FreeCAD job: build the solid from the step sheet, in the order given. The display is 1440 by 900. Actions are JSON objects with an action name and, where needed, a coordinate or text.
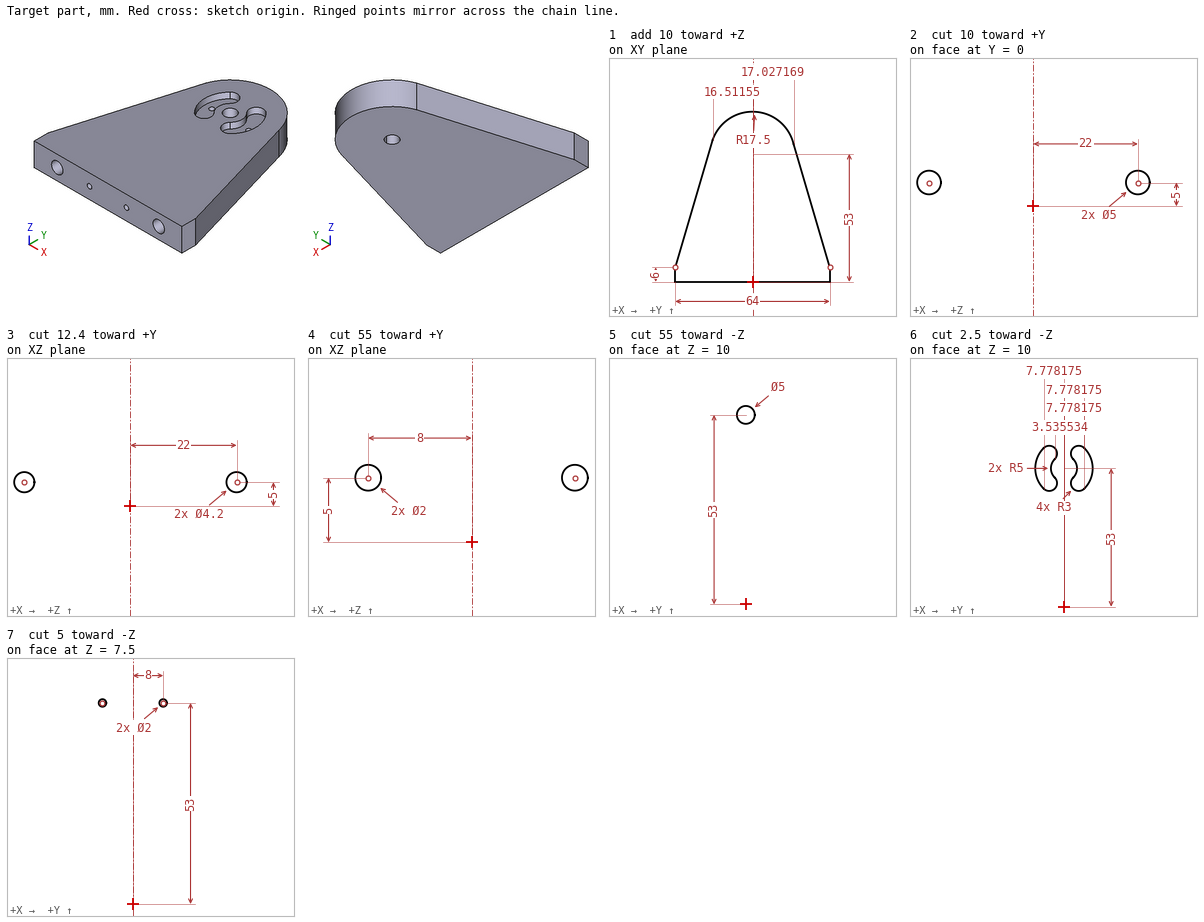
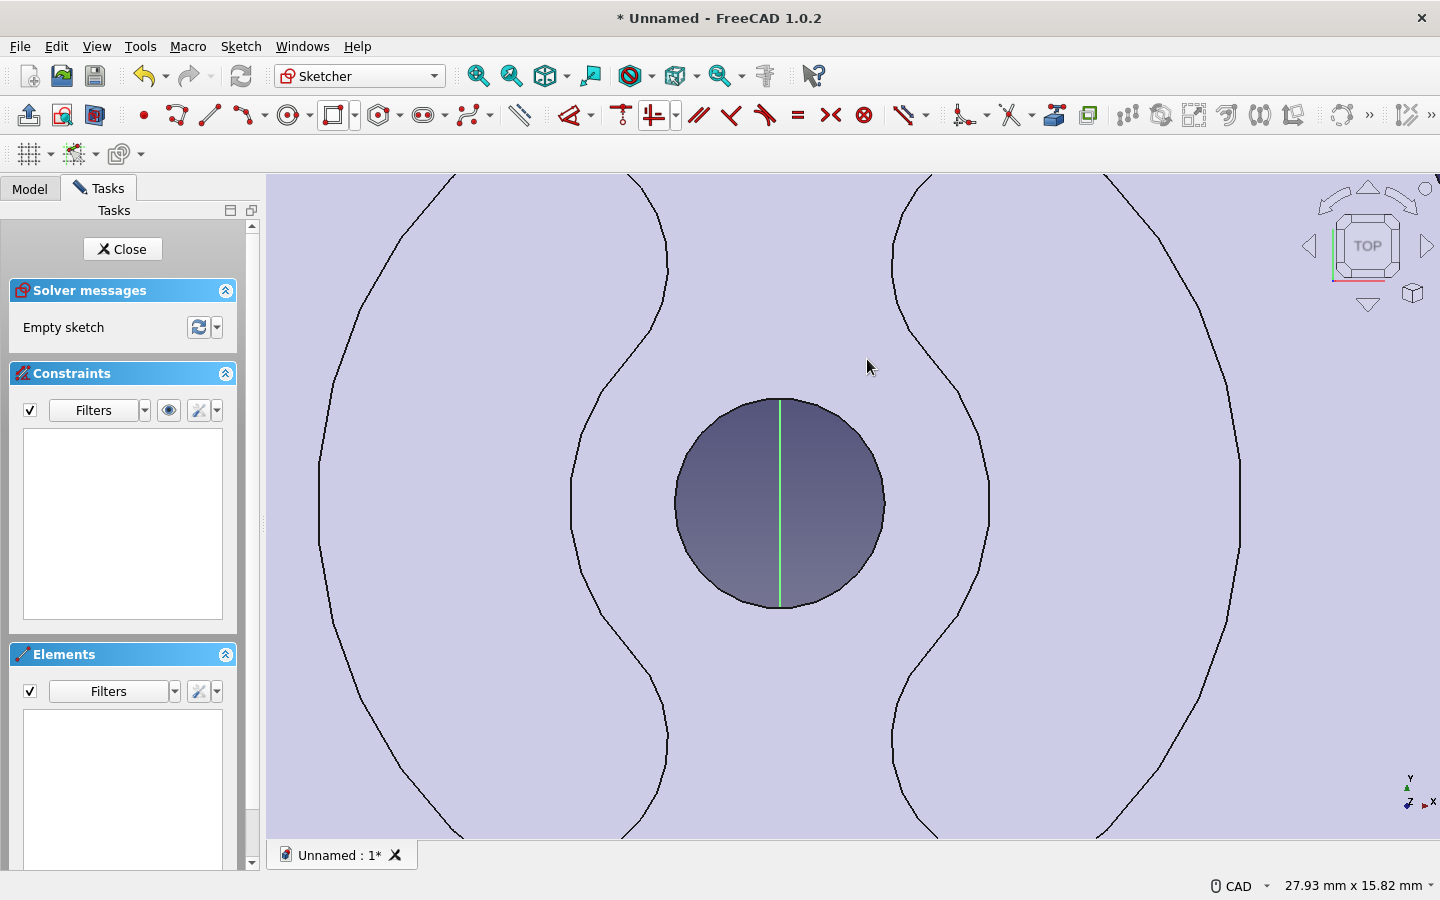
{"action": "left_click", "coordinate": [288, 116]}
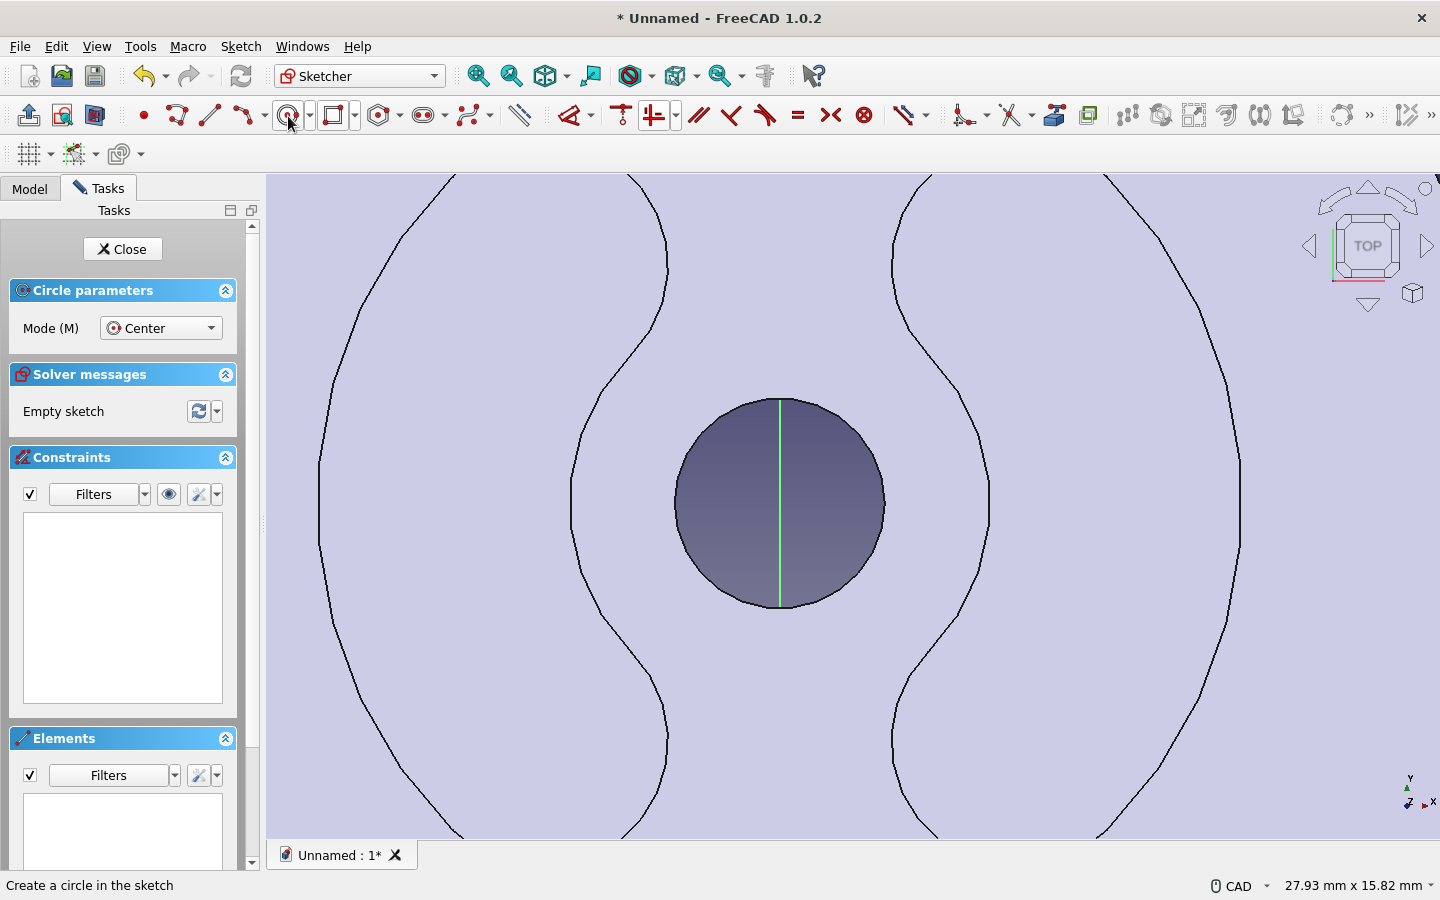
{"action": "left_click", "coordinate": [1116, 503]}
{"action": "mouse_move", "coordinate": [1146, 474]}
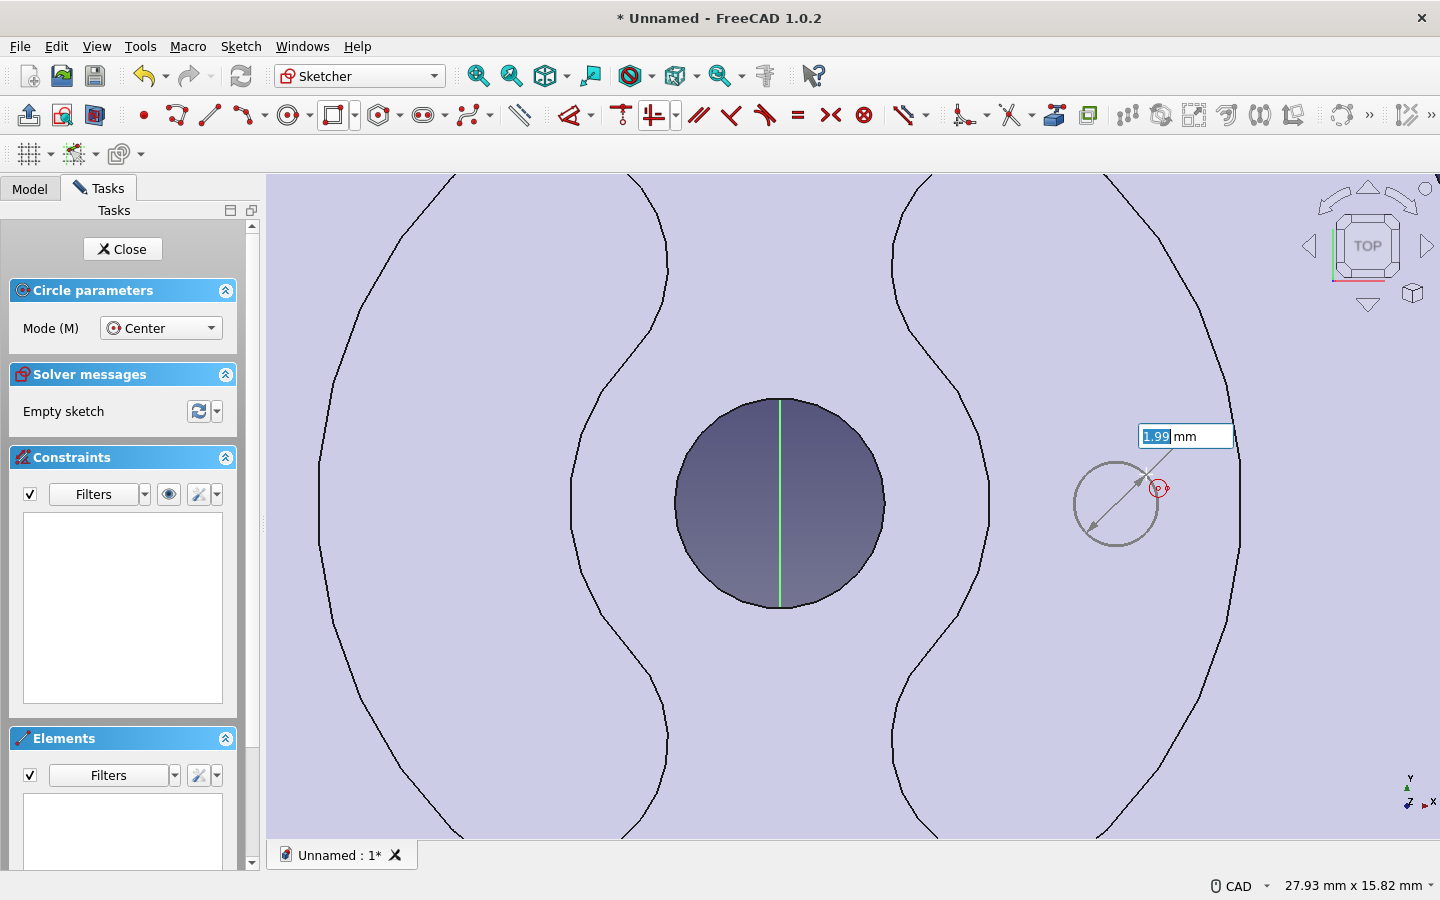
{"action": "type", "text": "2"}
{"action": "key", "text": "Return"}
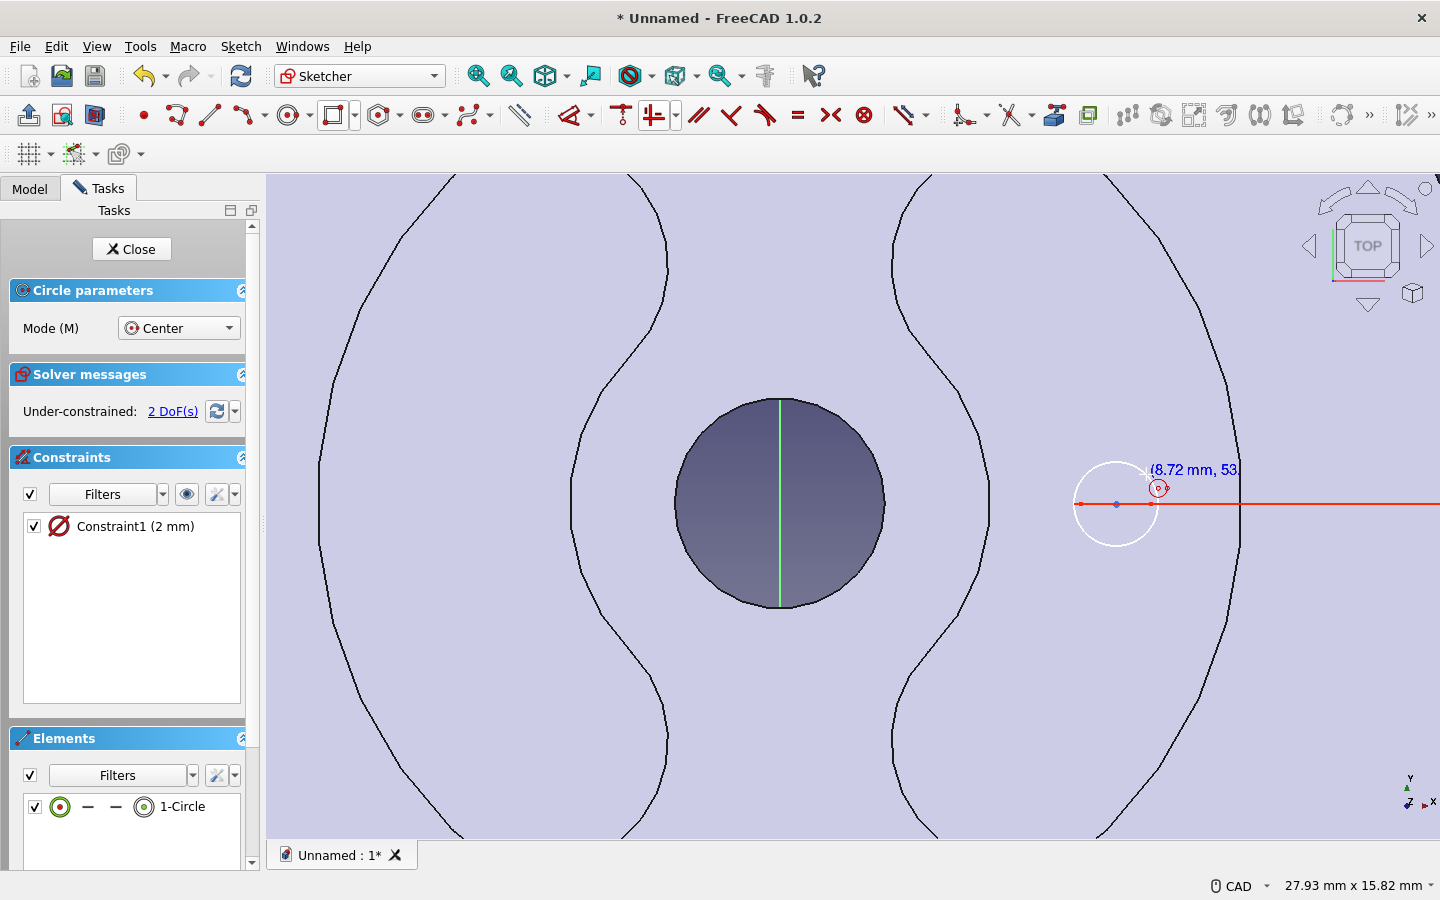
{"action": "left_click", "coordinate": [443, 503]}
{"action": "mouse_move", "coordinate": [473, 474]}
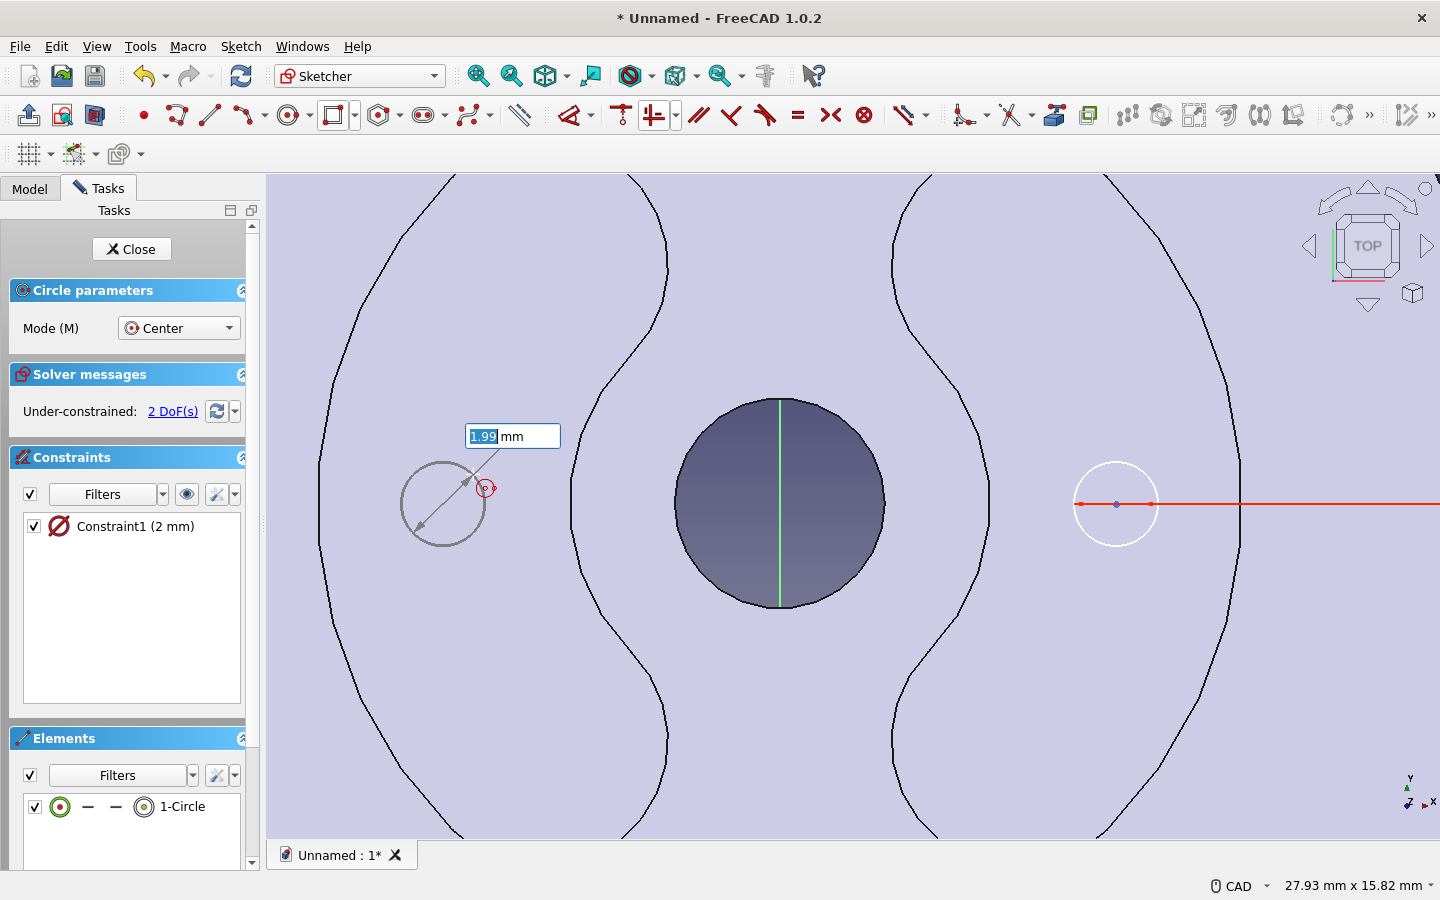
{"action": "type", "text": "2"}
{"action": "key", "text": "Return"}
{"action": "key", "text": "Escape"}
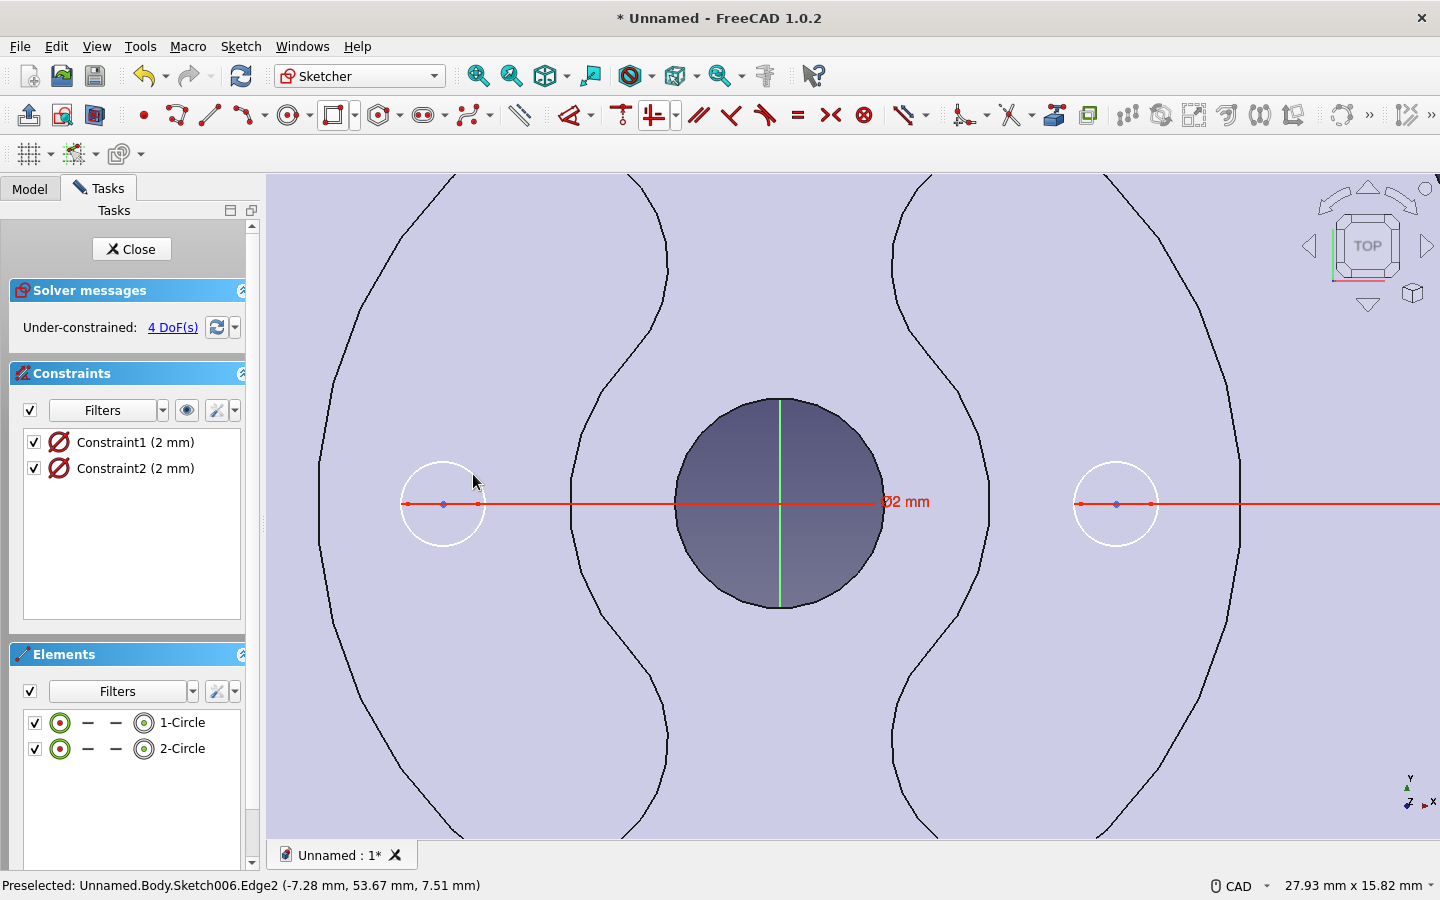
{"action": "left_click", "coordinate": [1116, 504]}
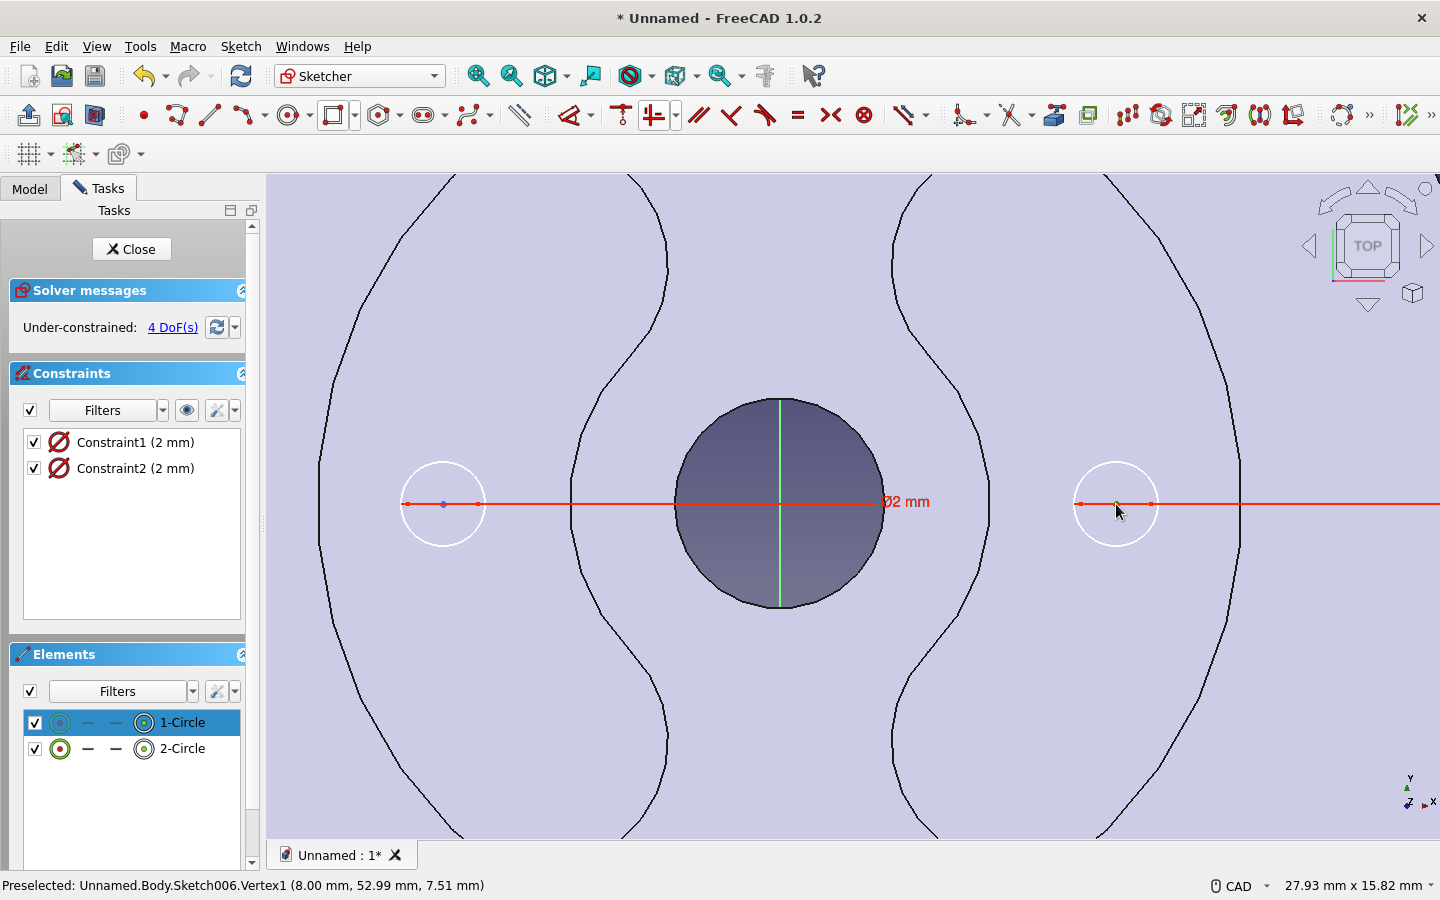
{"action": "left_click", "coordinate": [443, 504]}